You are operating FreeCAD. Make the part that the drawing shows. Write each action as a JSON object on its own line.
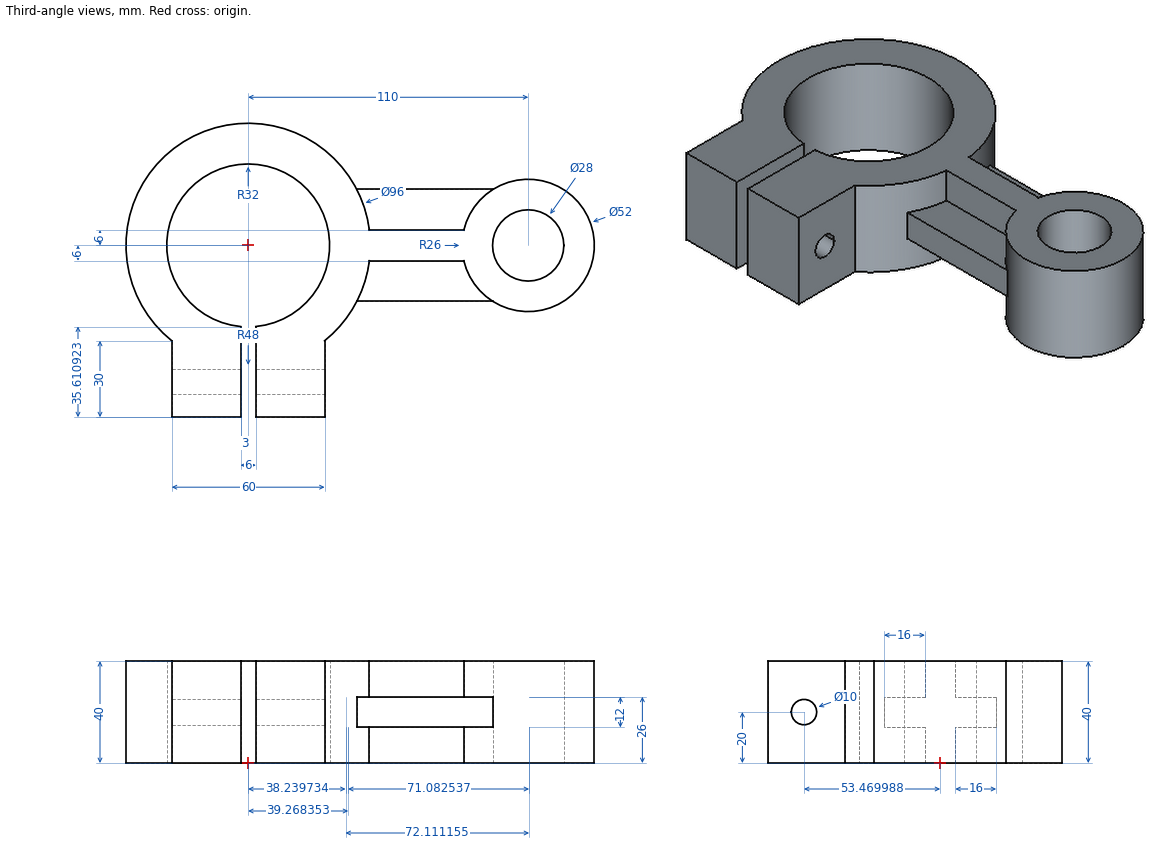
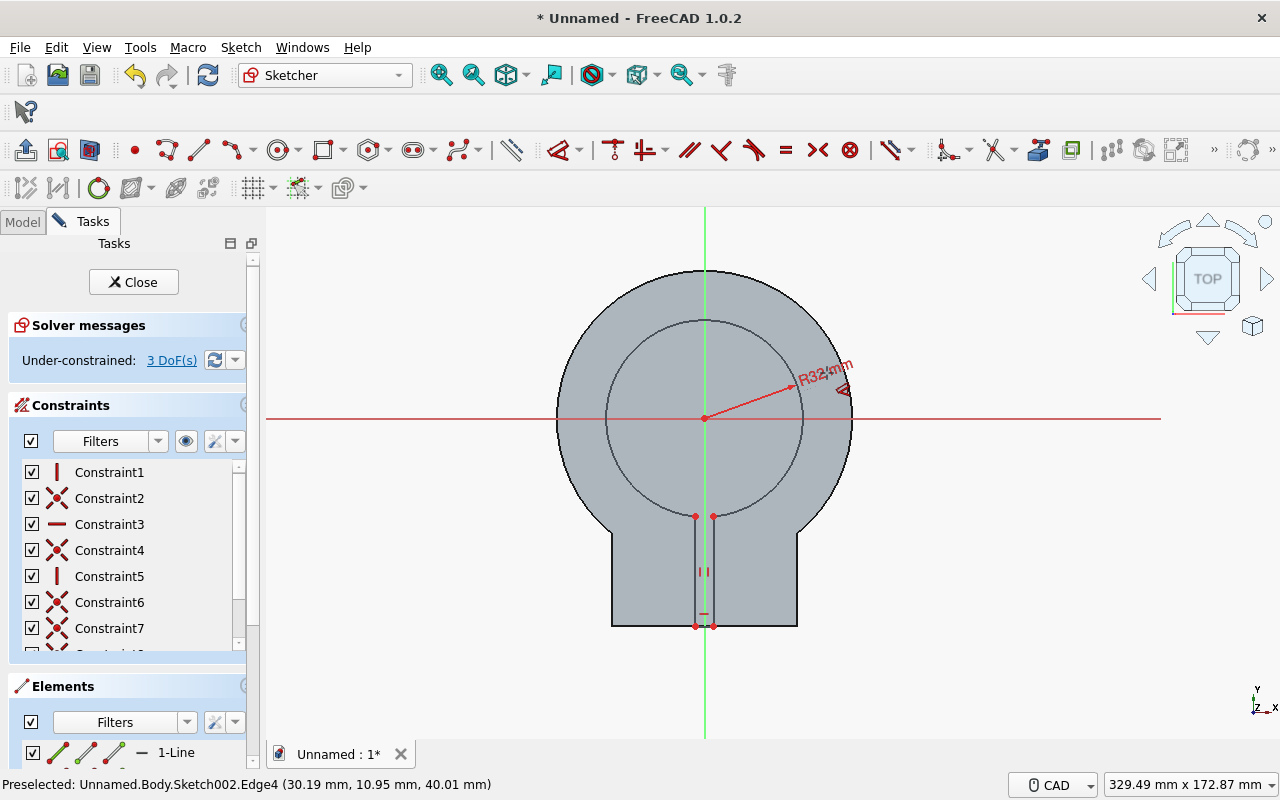
{"action": "scroll", "coordinate": [705, 627], "scroll_direction": "up", "scroll_amount": 4}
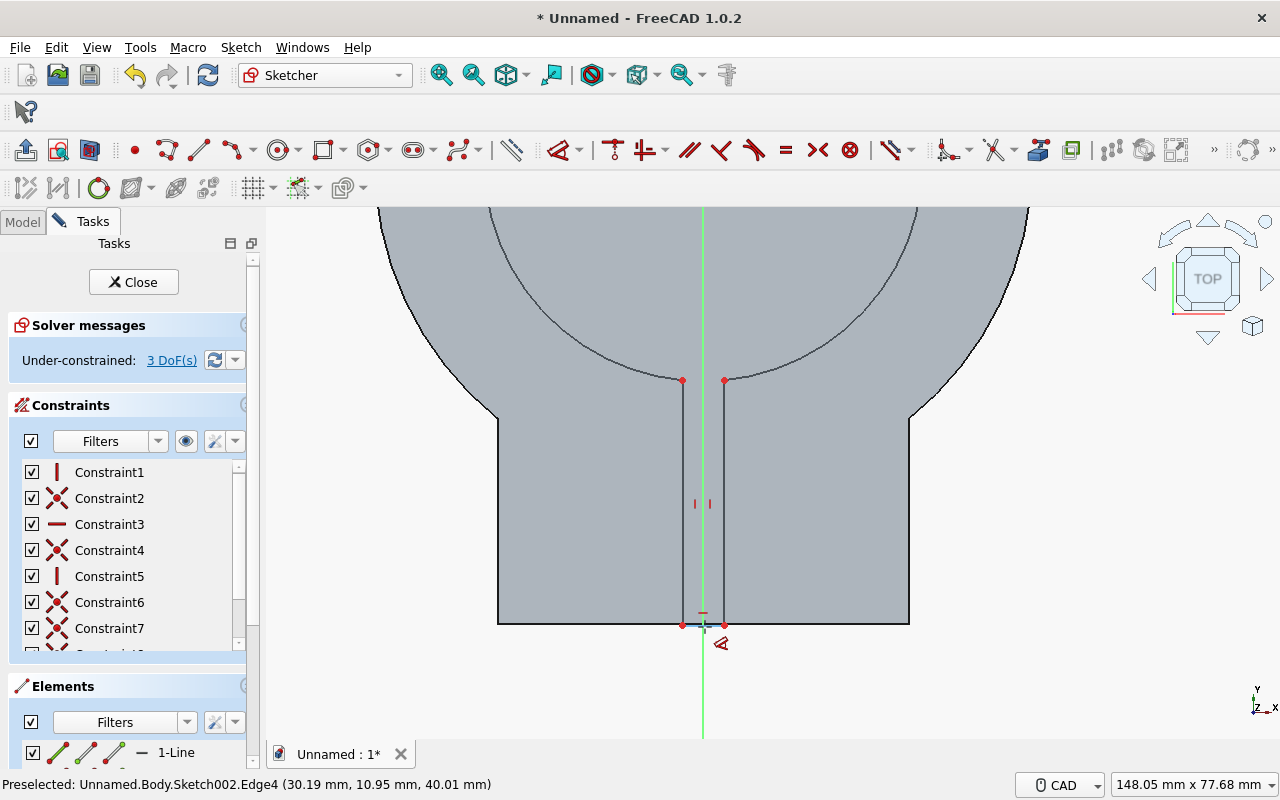
{"action": "left_click", "coordinate": [703, 626]}
{"action": "left_click", "coordinate": [689, 660]}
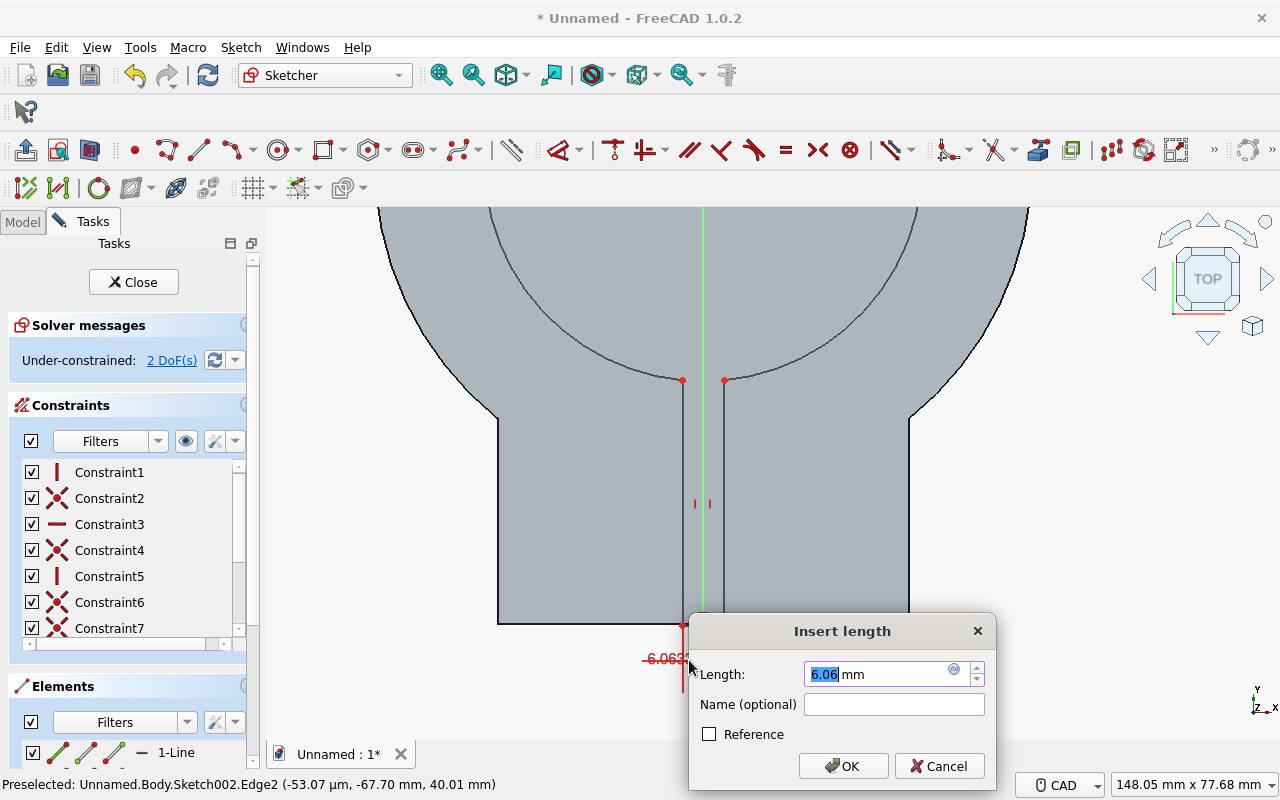
{"action": "type", "text": "6"}
{"action": "key", "text": "Return"}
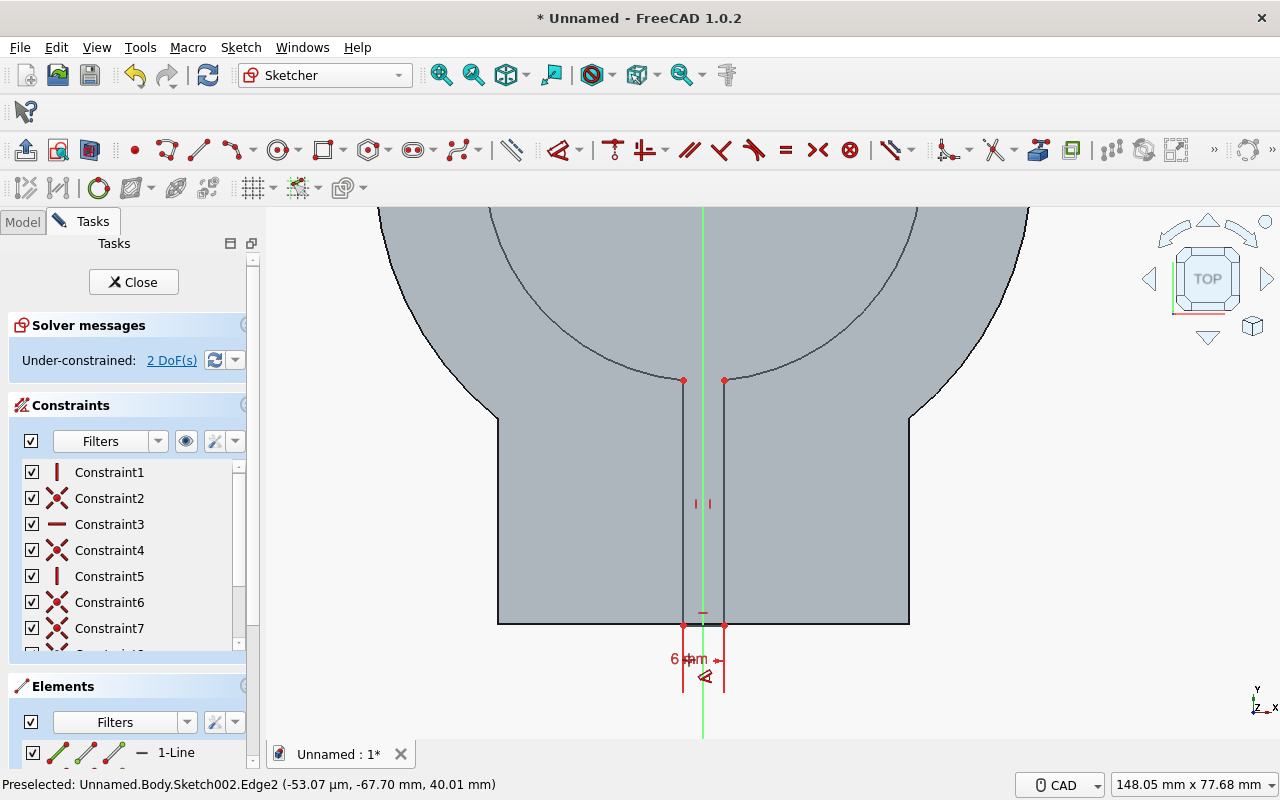
{"action": "scroll", "coordinate": [683, 380], "scroll_direction": "up", "scroll_amount": 4}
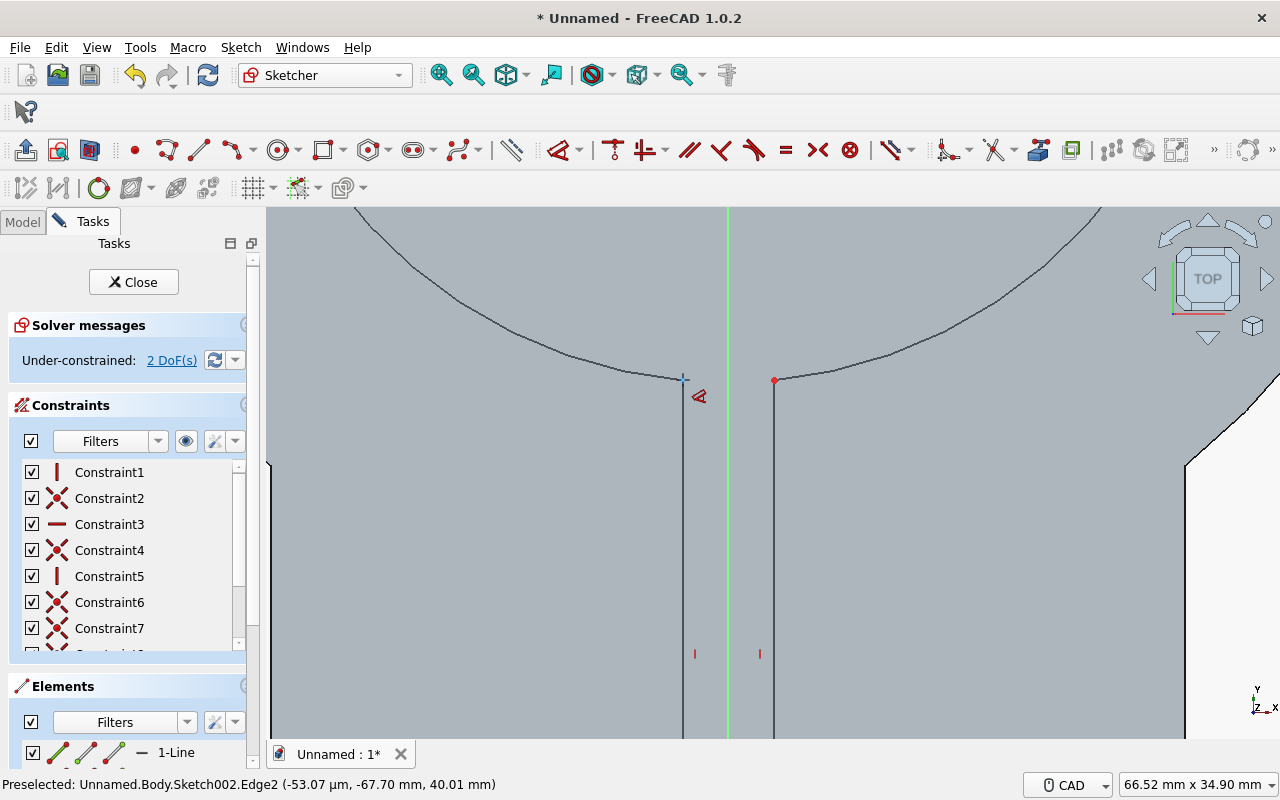
{"action": "left_click", "coordinate": [683, 380]}
{"action": "left_click", "coordinate": [705, 414]}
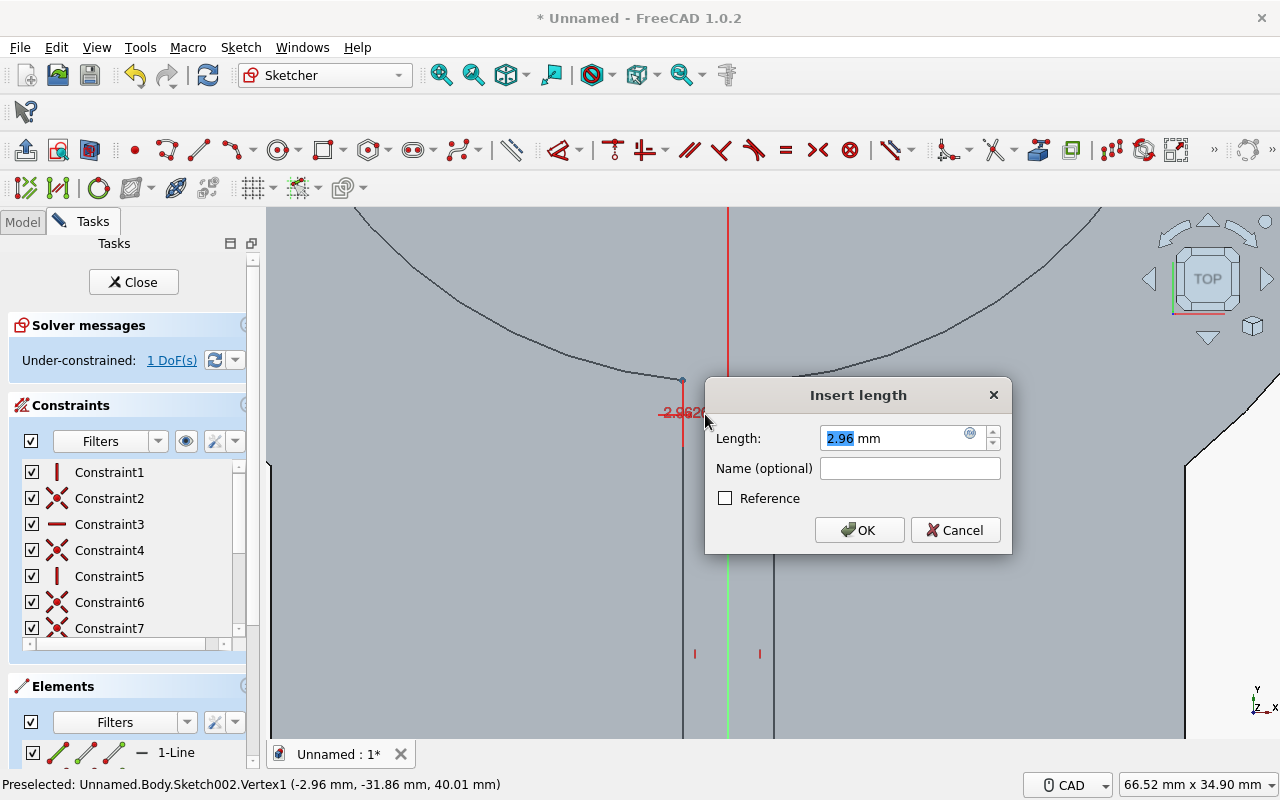
{"action": "type", "text": "3"}
{"action": "key", "text": "Return"}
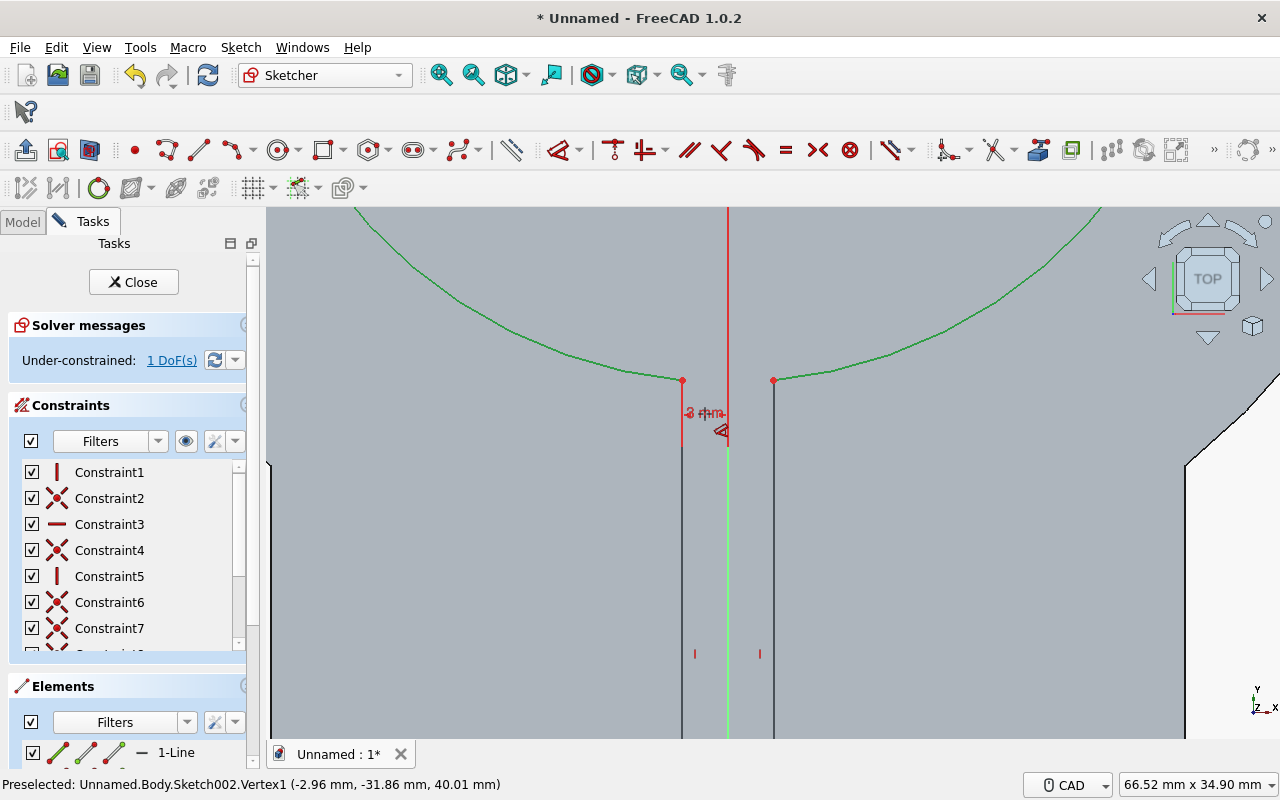
{"action": "scroll", "coordinate": [699, 551], "scroll_direction": "down", "scroll_amount": 8}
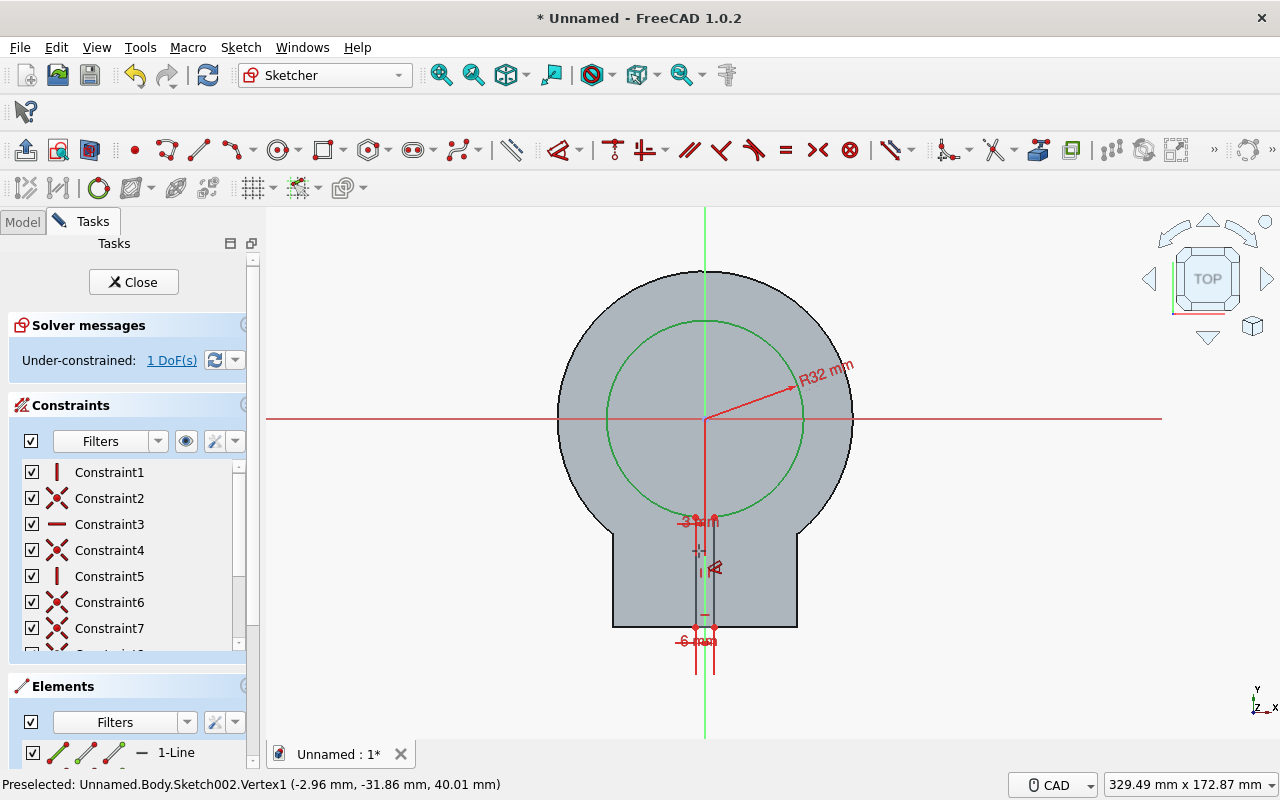
{"action": "scroll", "coordinate": [696, 550], "scroll_direction": "up", "scroll_amount": 3}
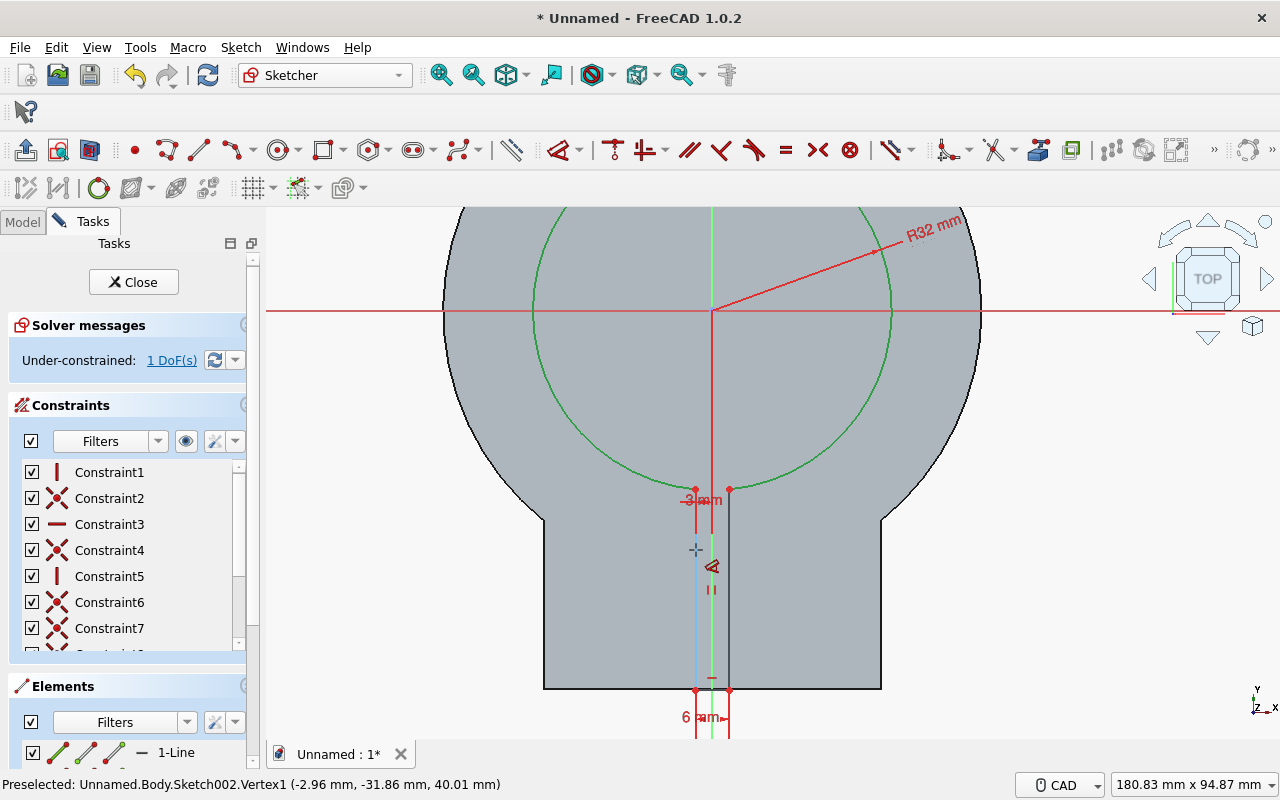
{"action": "left_click", "coordinate": [696, 550]}
{"action": "left_click", "coordinate": [662, 590]}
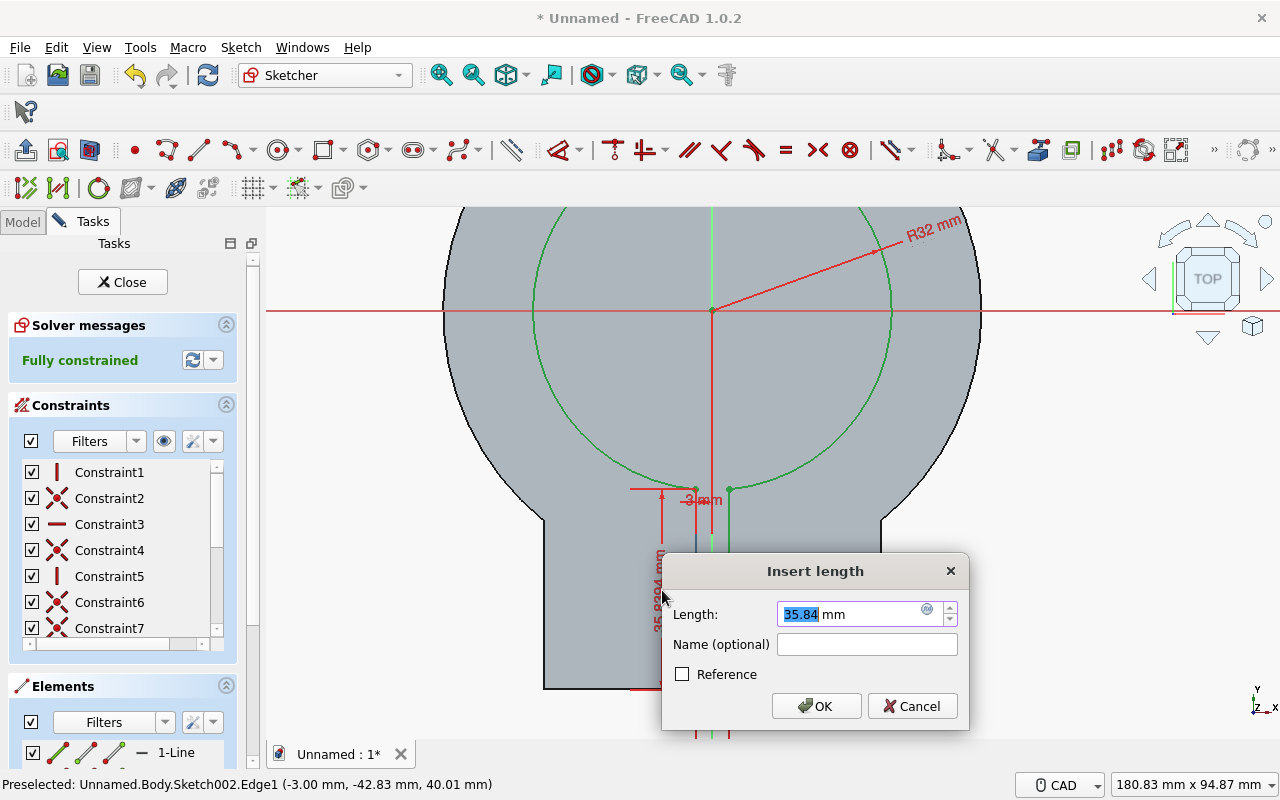
{"action": "type", "text": "35.610923"}
{"action": "key", "text": "Return"}
{"action": "key", "text": "Escape"}